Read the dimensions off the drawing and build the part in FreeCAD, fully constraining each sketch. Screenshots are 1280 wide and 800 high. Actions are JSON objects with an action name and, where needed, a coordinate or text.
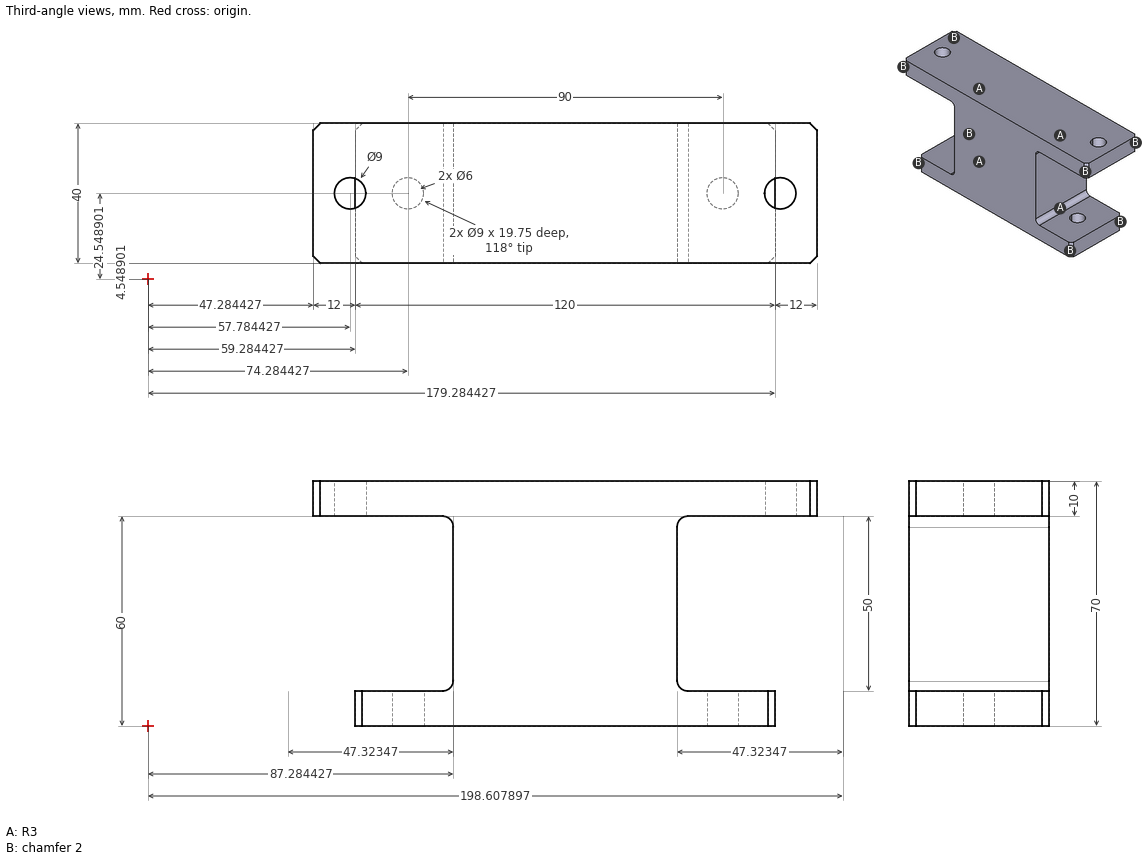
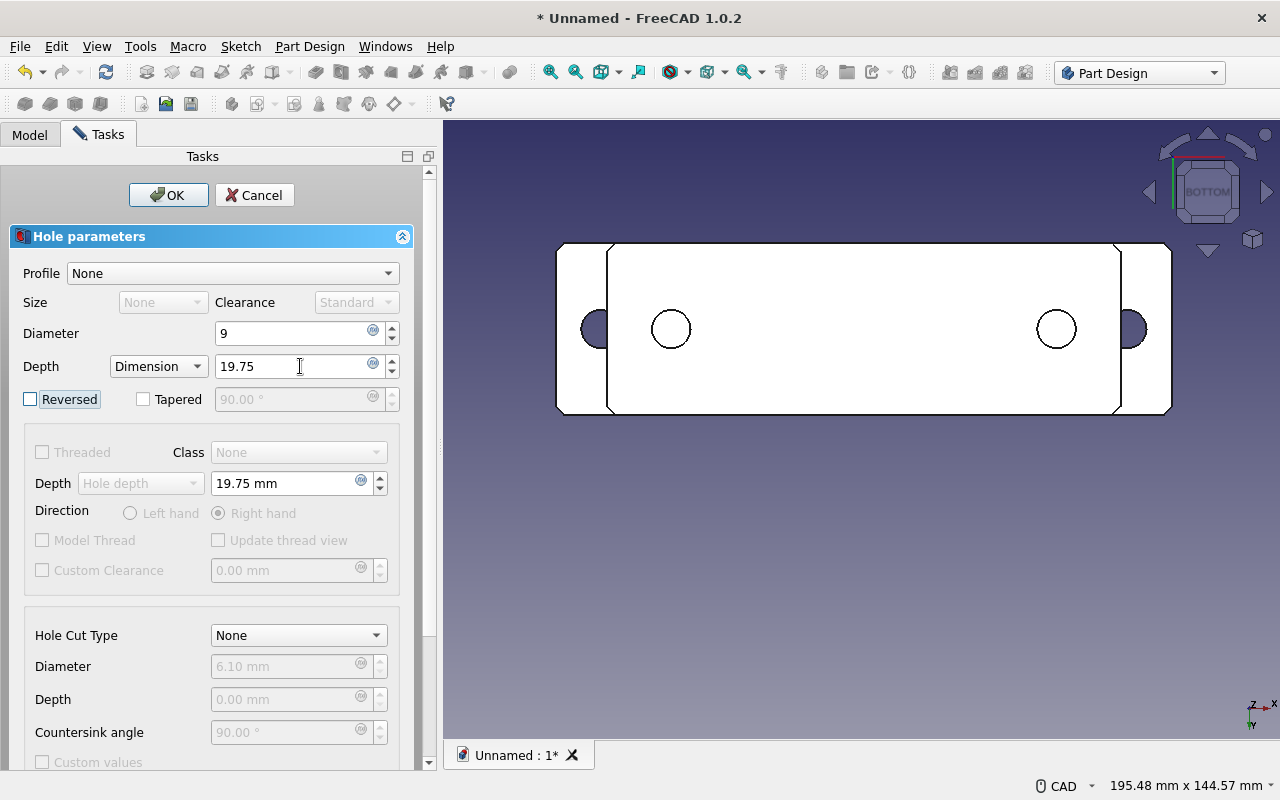
{"action": "left_click", "coordinate": [169, 195]}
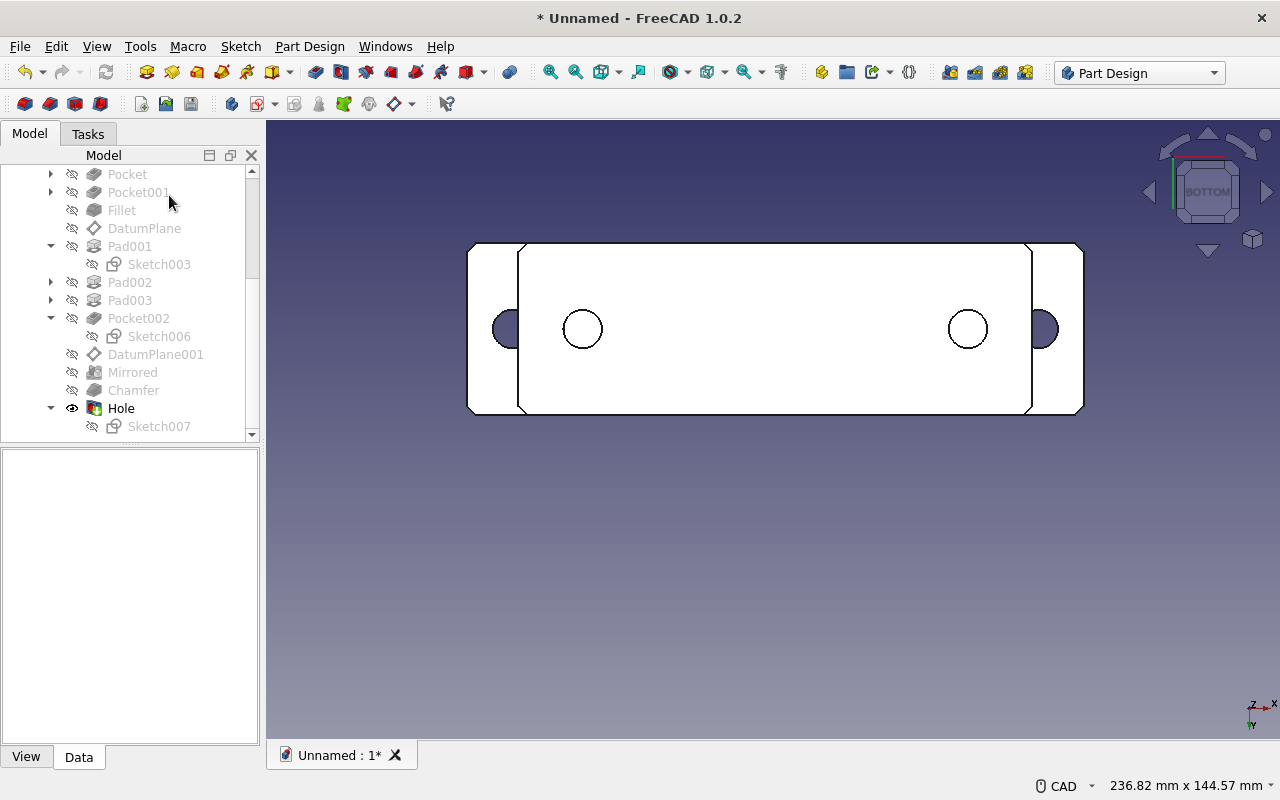
{"action": "key", "text": "0"}